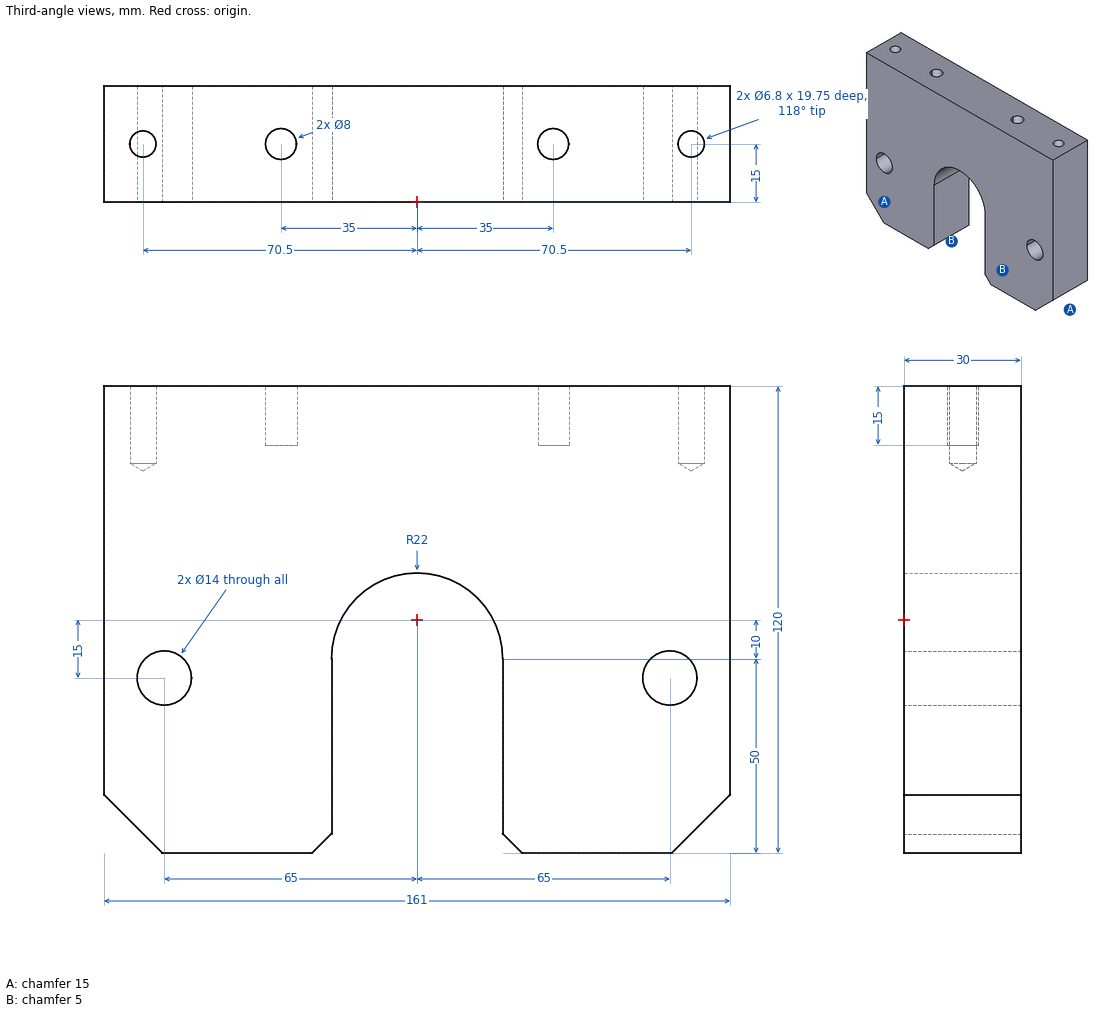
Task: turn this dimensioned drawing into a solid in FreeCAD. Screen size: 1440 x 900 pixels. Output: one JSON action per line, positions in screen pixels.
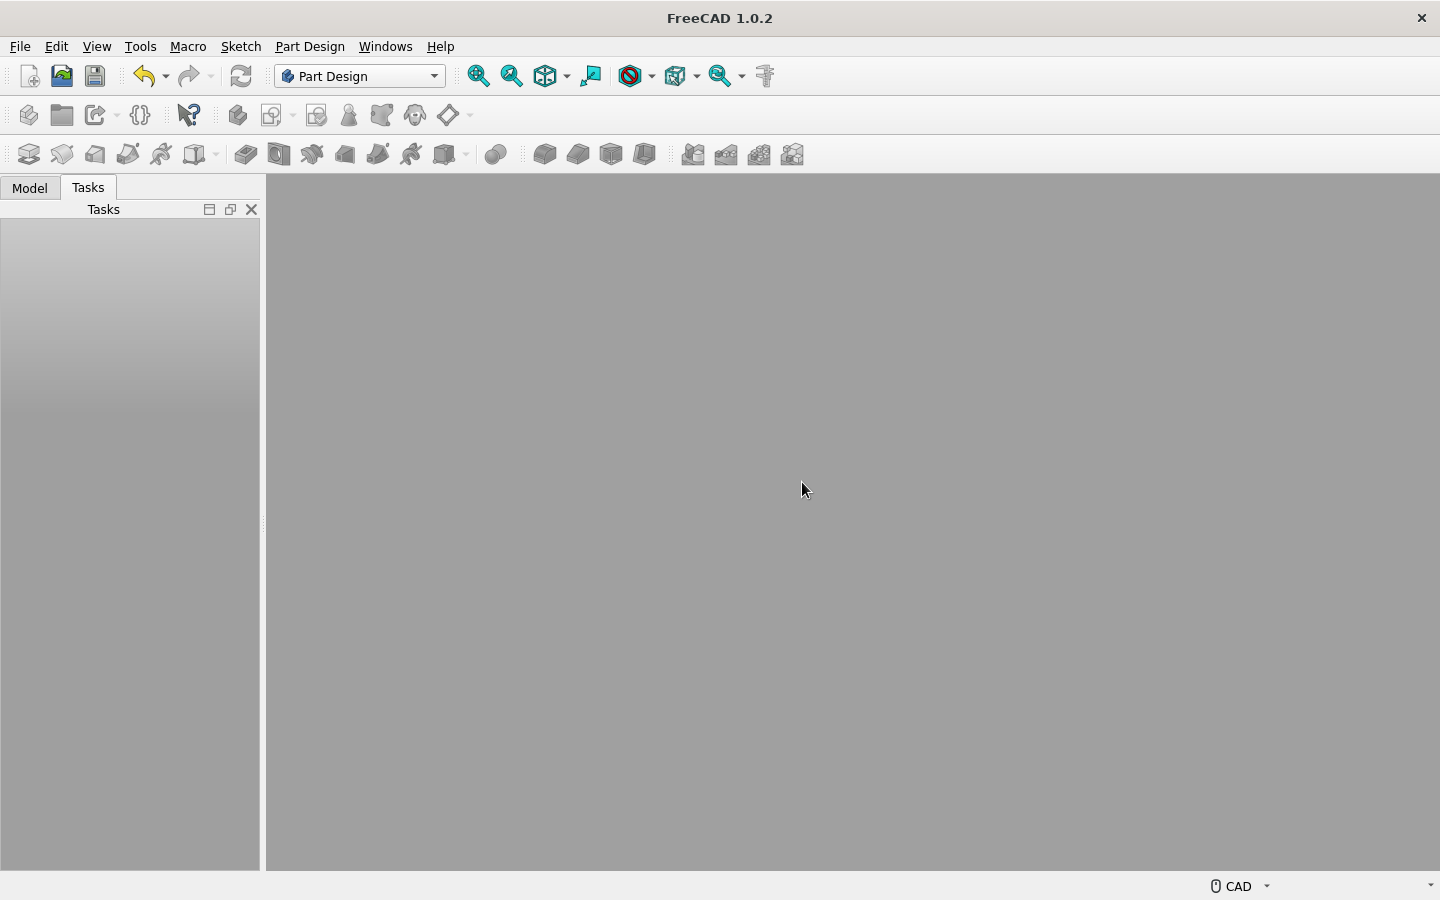
{"action": "left_click", "coordinate": [29, 76]}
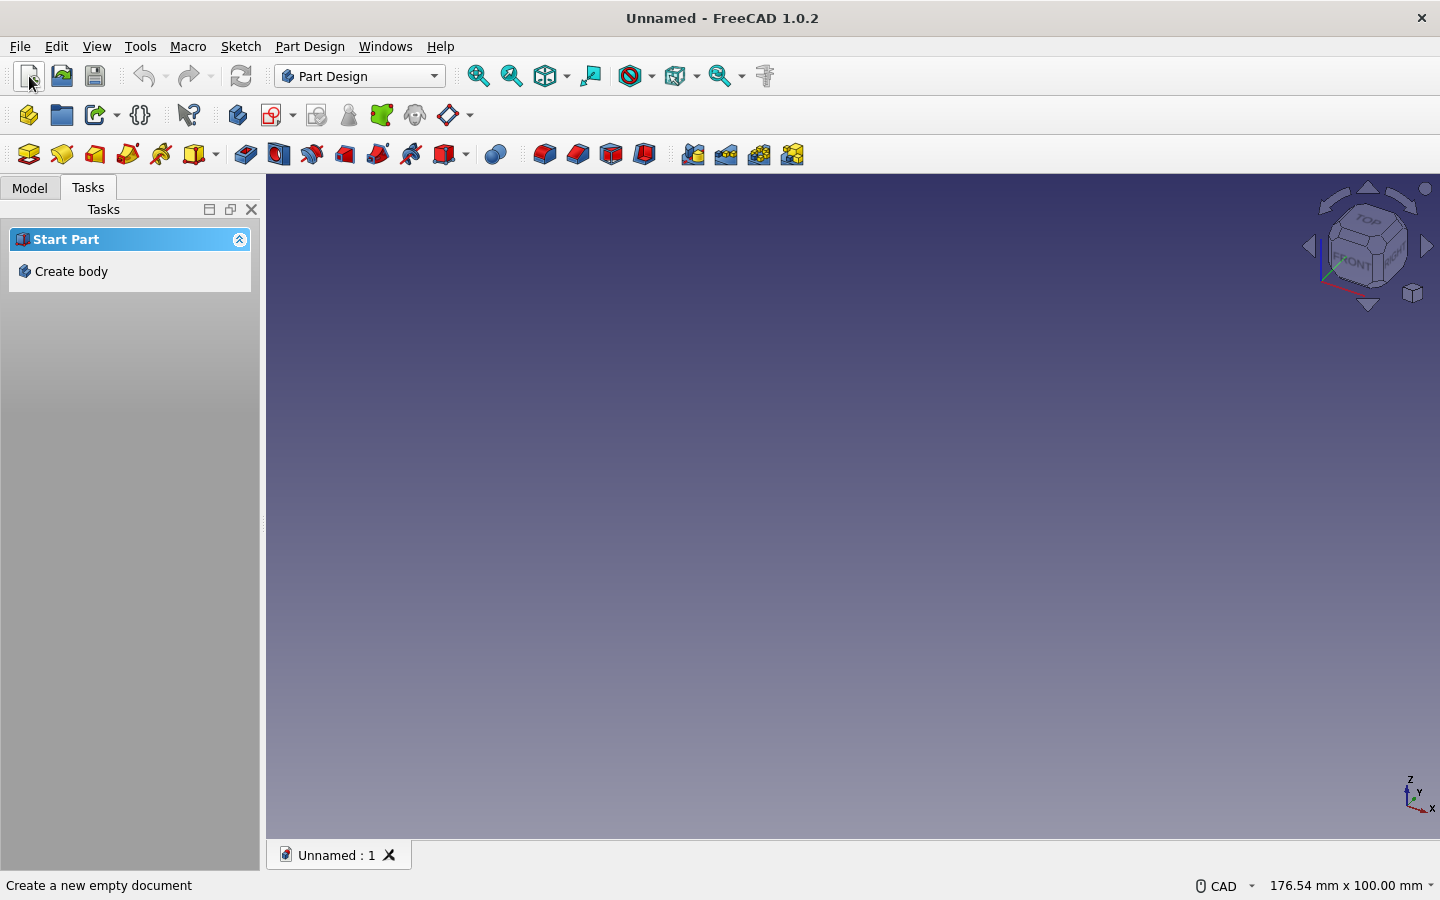
{"action": "left_click", "coordinate": [270, 116]}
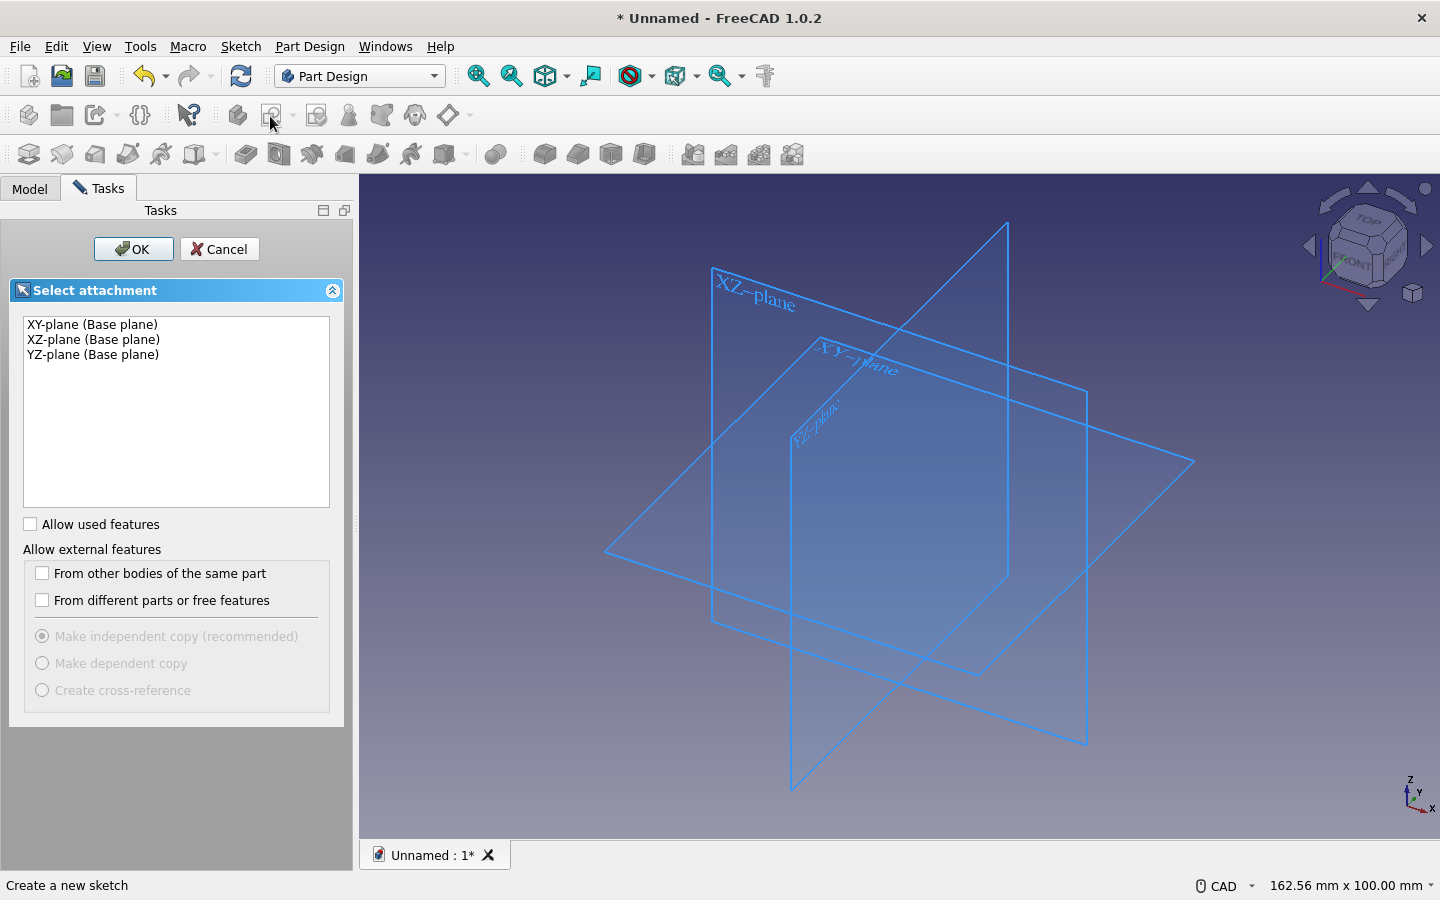
{"action": "left_click", "coordinate": [84, 340]}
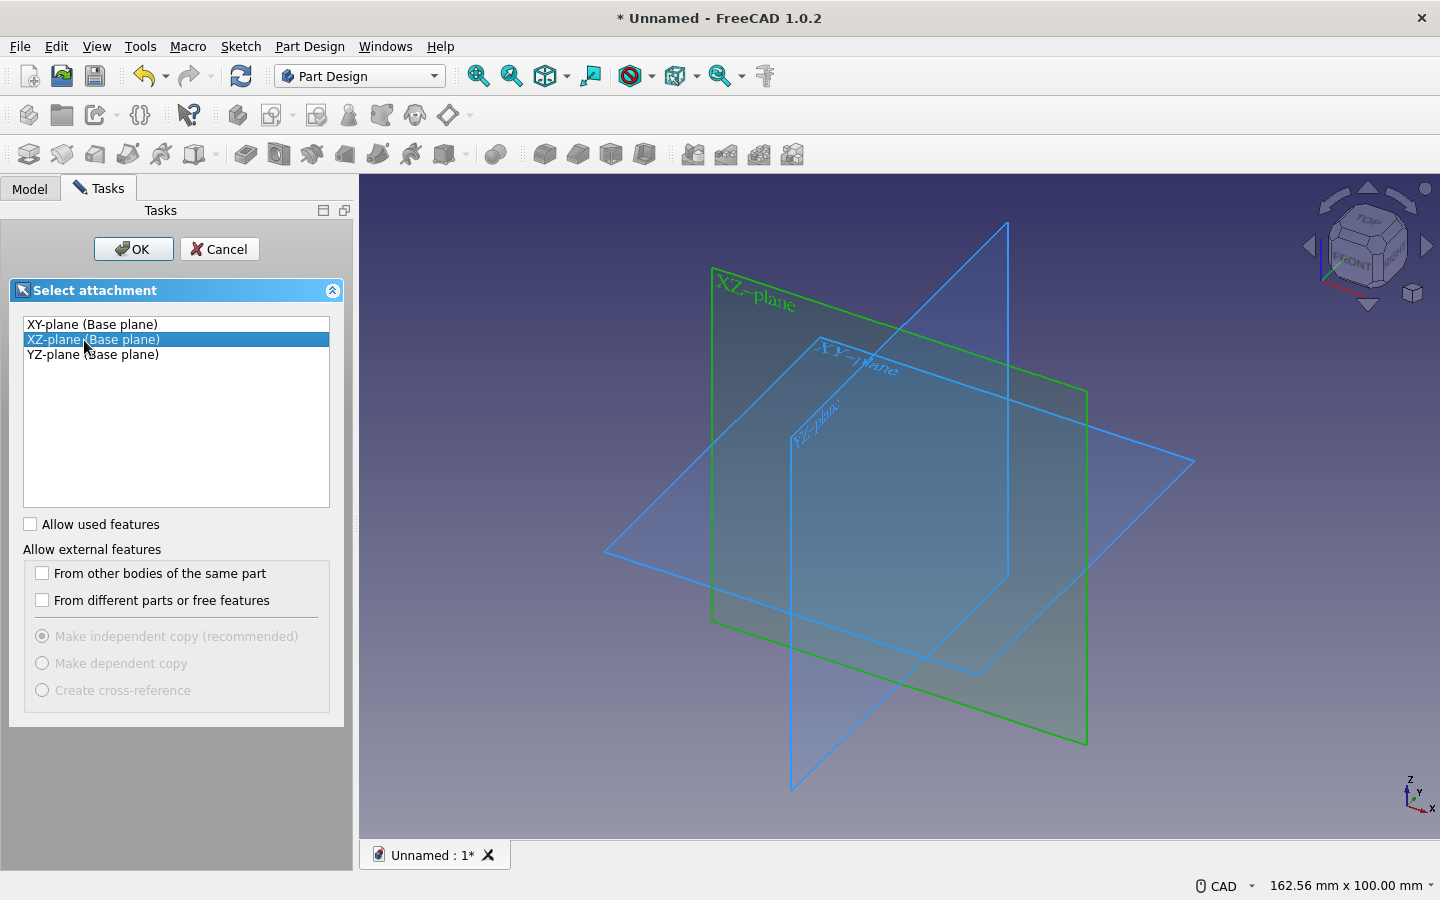
{"action": "left_click", "coordinate": [134, 249]}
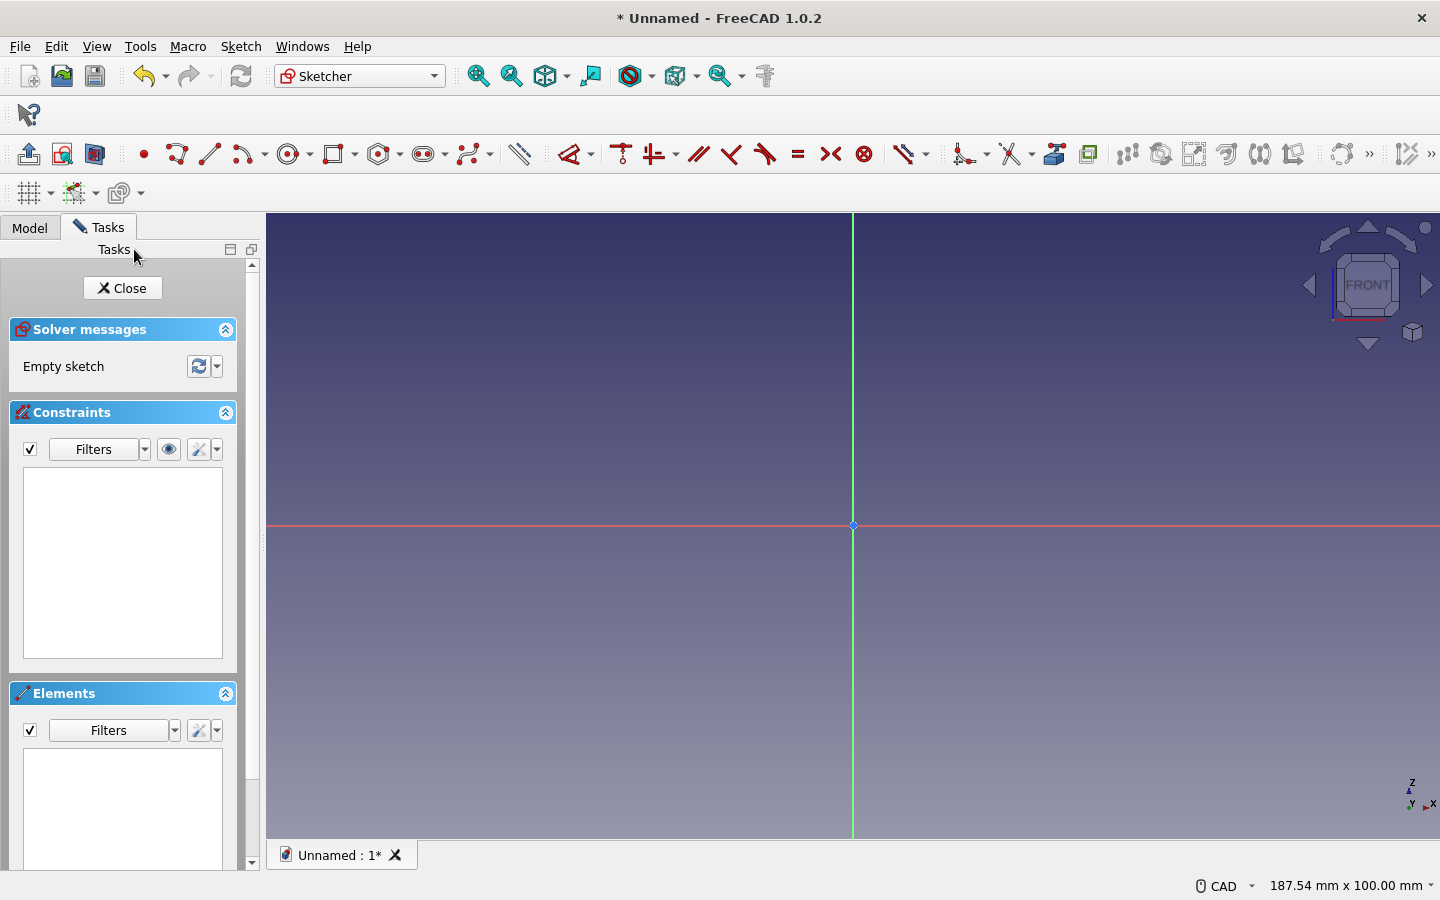
{"action": "scroll", "coordinate": [701, 526], "scroll_direction": "down", "scroll_amount": 3}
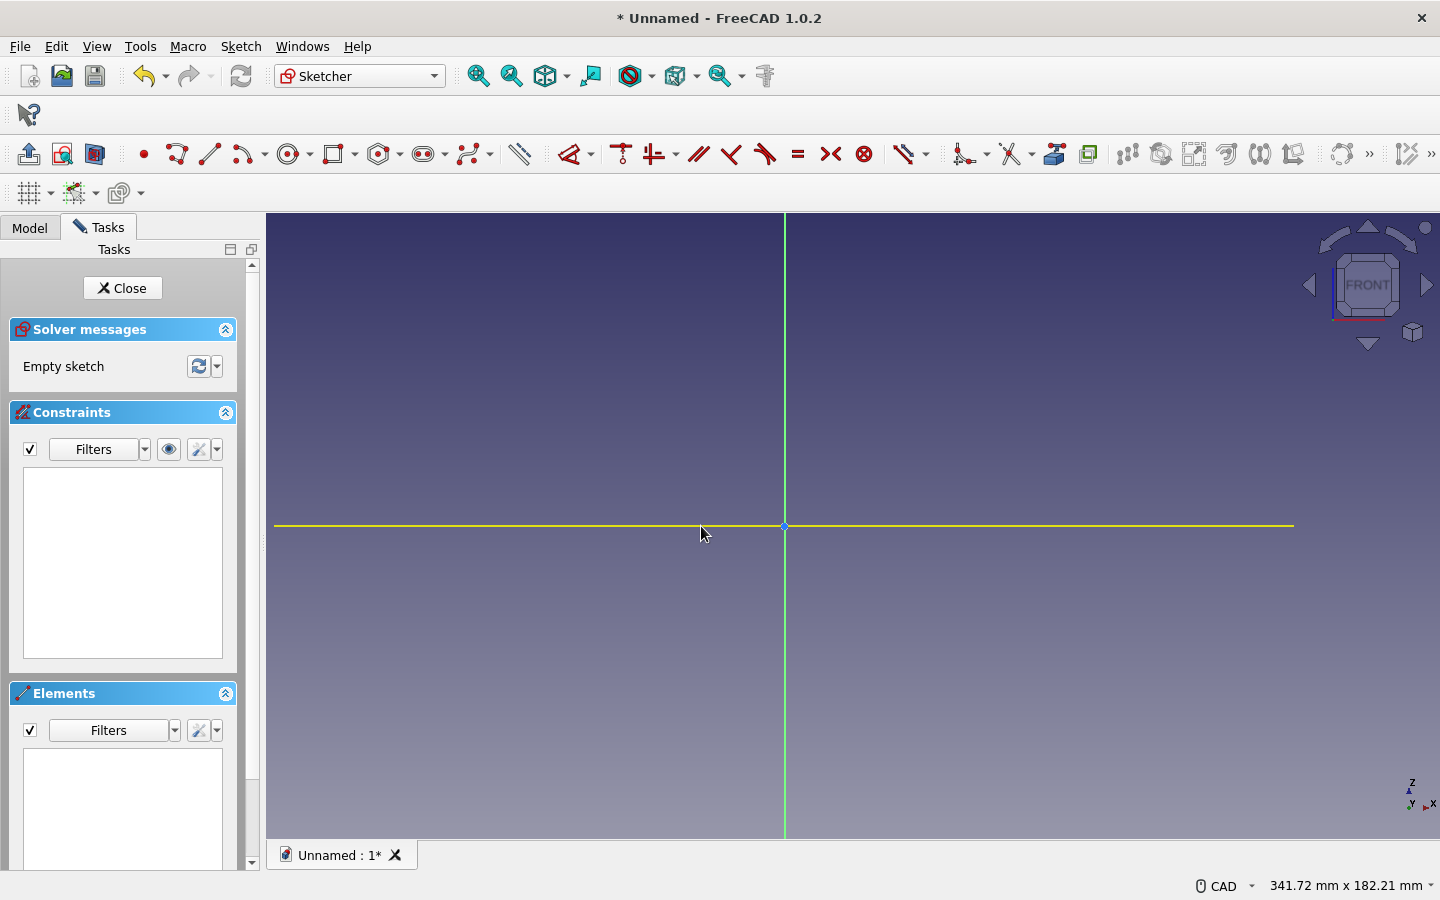
{"action": "key", "text": "g v"}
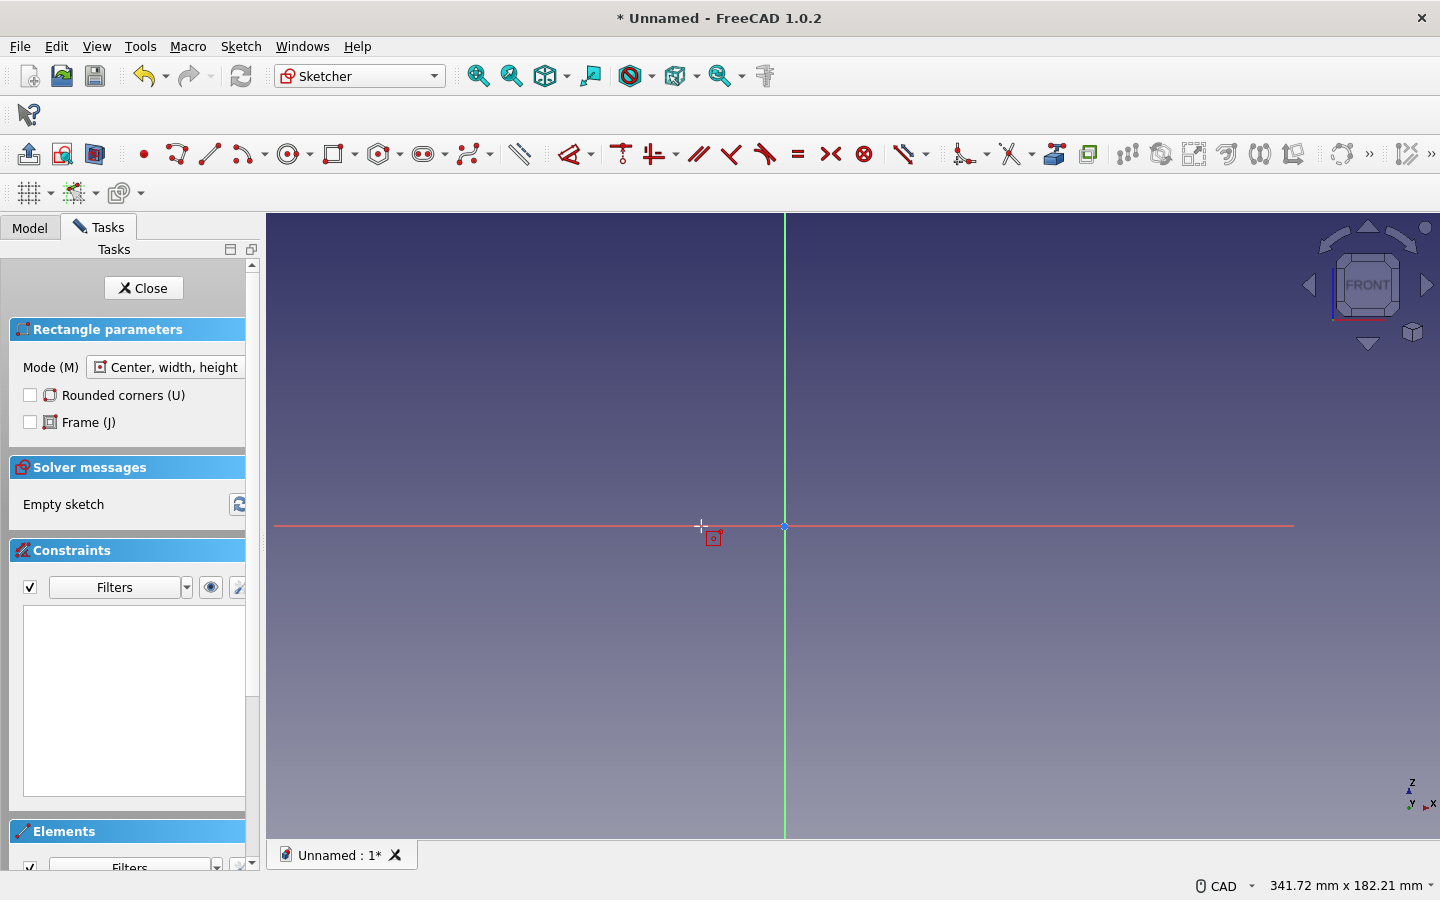
{"action": "left_click", "coordinate": [785, 526]}
{"action": "left_click", "coordinate": [1061, 320]}
{"action": "key", "text": "Escape"}